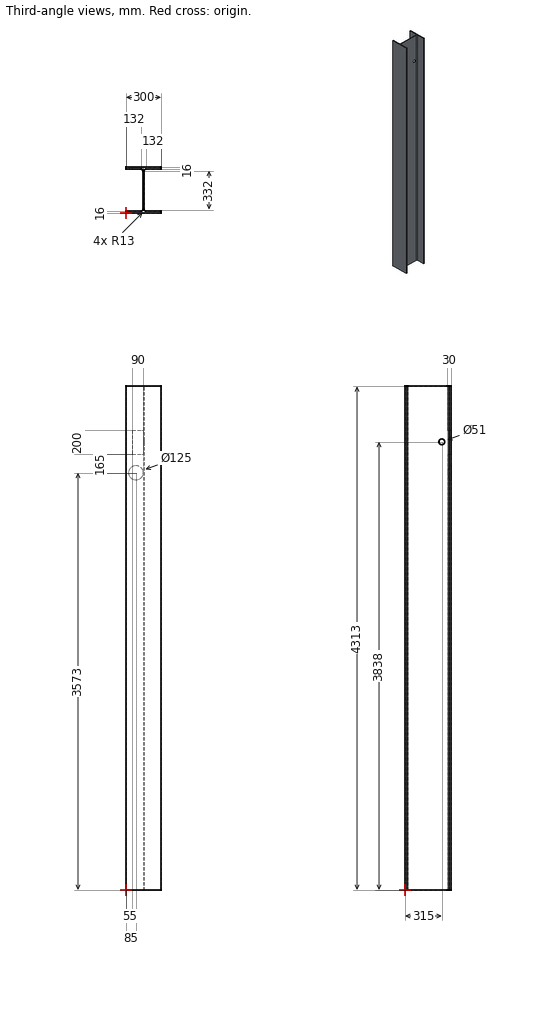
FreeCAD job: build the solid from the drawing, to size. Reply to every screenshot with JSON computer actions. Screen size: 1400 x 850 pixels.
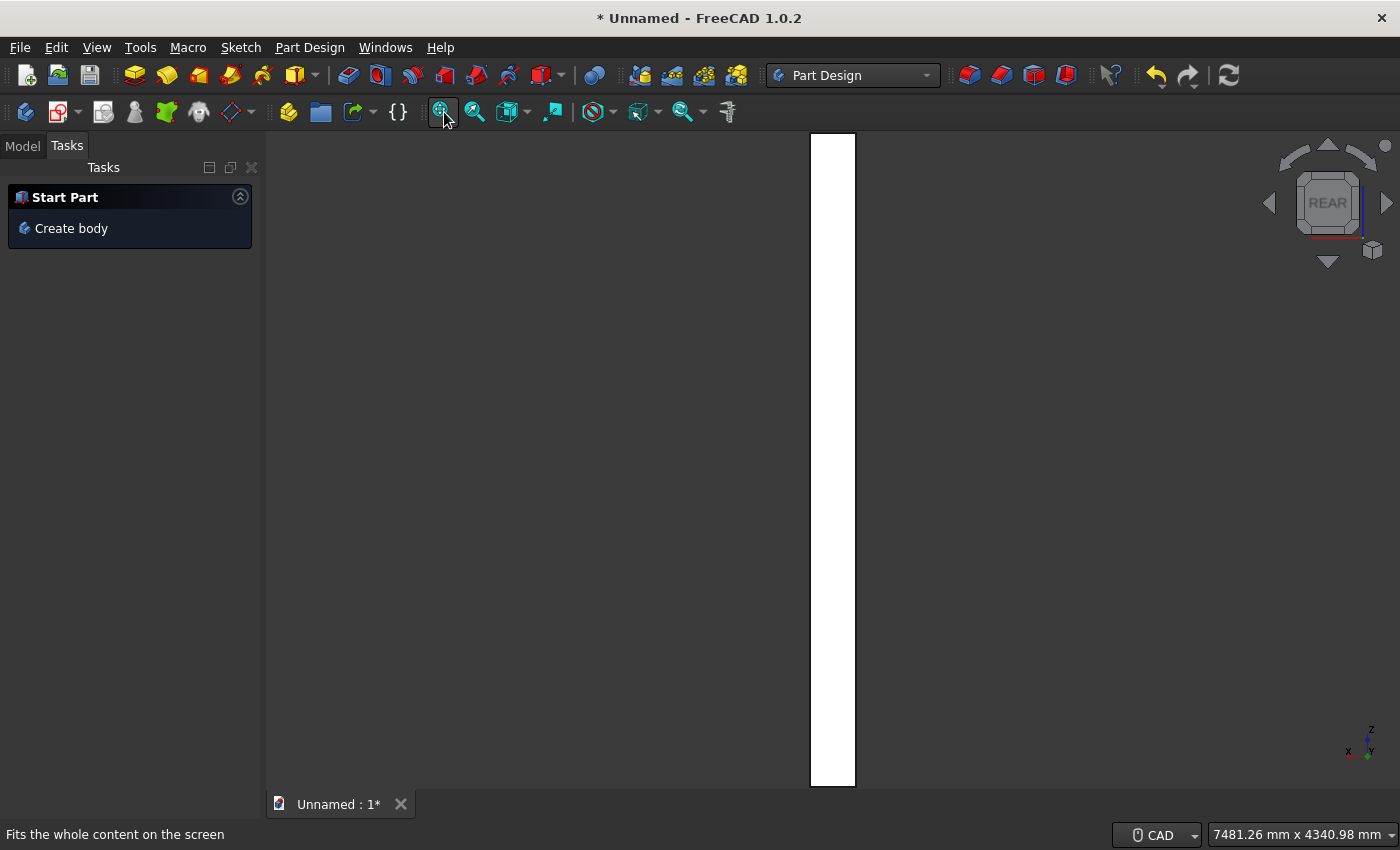
{"action": "left_click", "coordinate": [833, 179]}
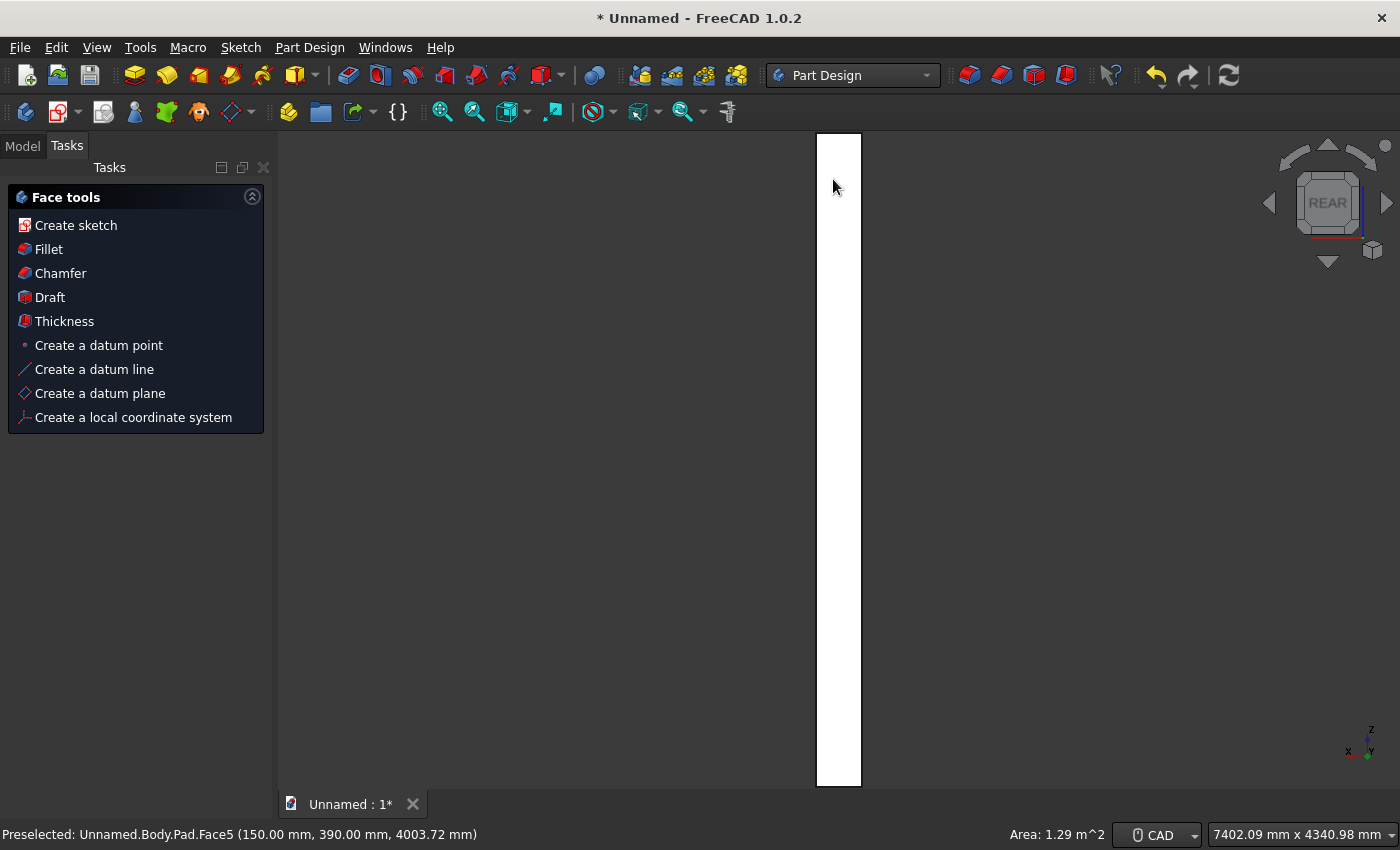
{"action": "left_click", "coordinate": [58, 112]}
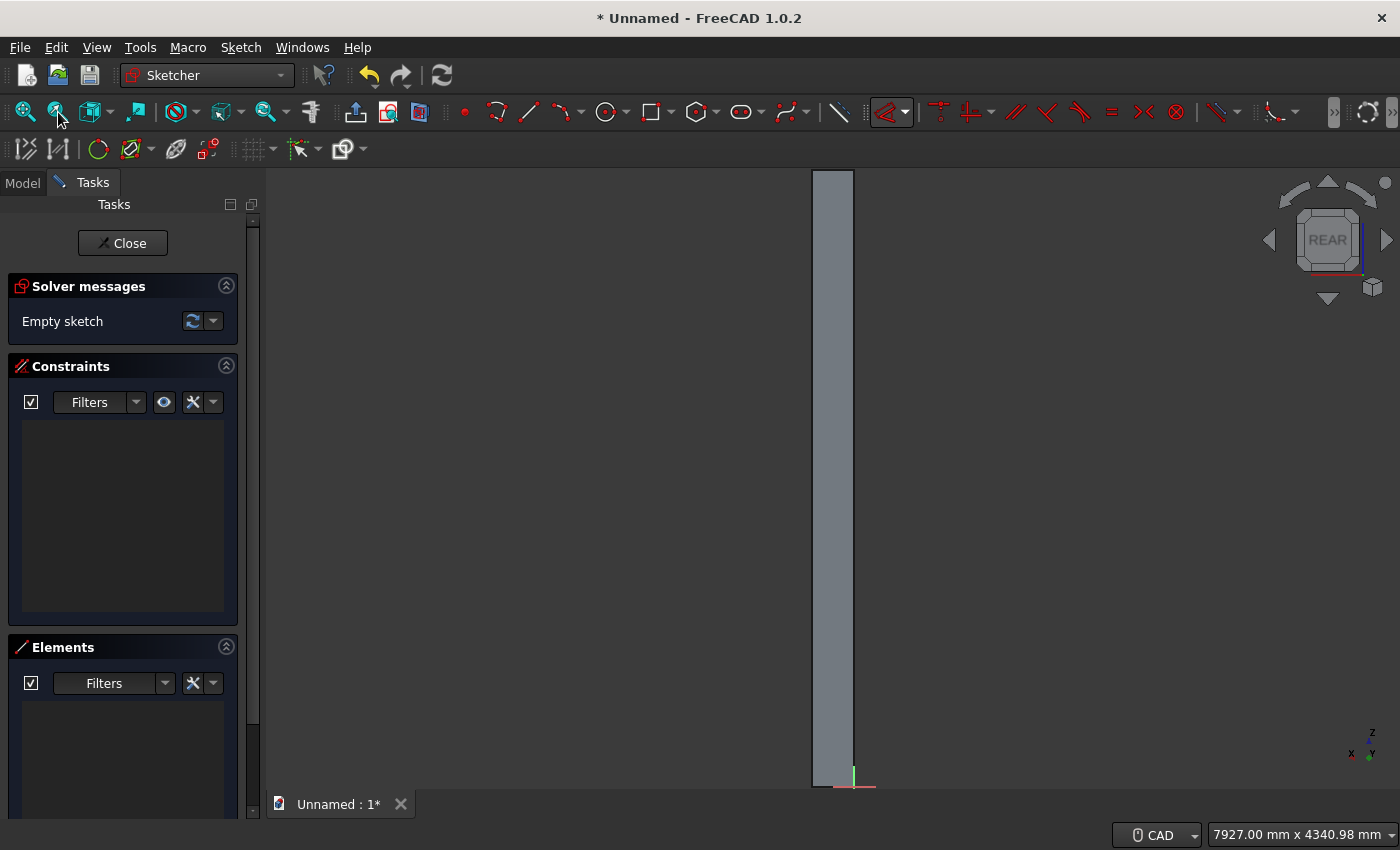
{"action": "scroll", "coordinate": [858, 210], "scroll_direction": "up", "scroll_amount": 9}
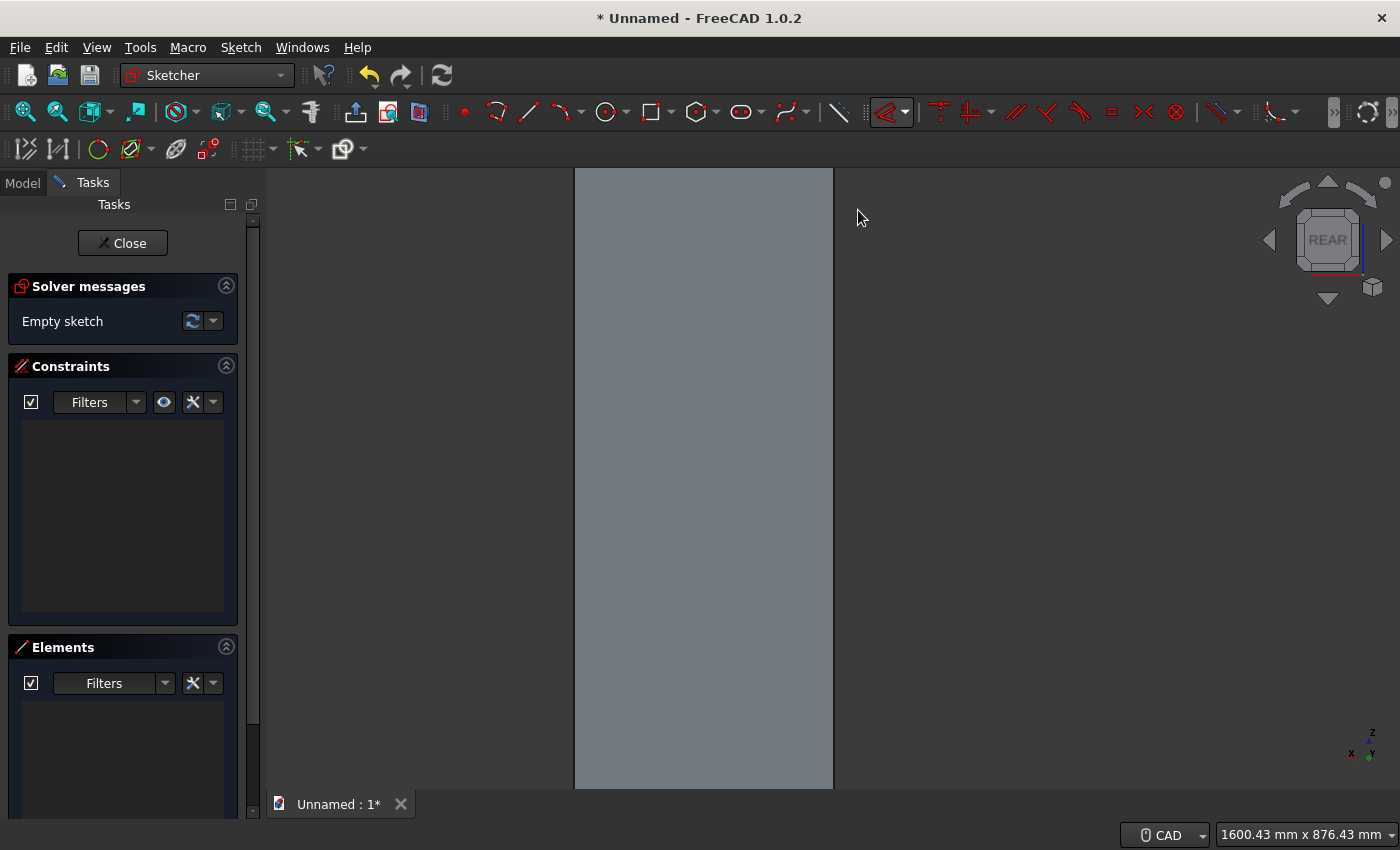
{"action": "left_click", "coordinate": [652, 112]}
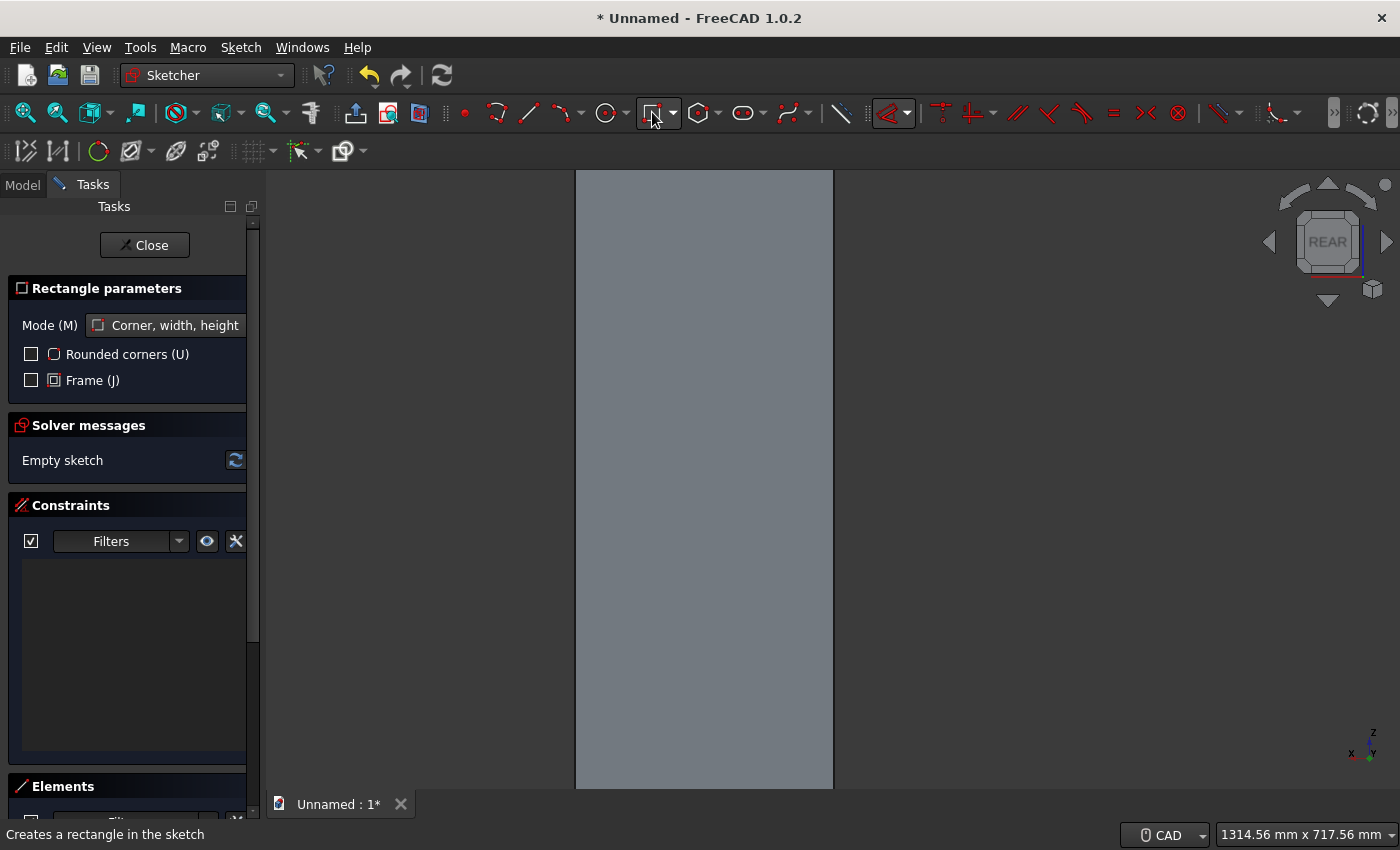
{"action": "left_click", "coordinate": [709, 294]}
{"action": "mouse_move", "coordinate": [786, 466]}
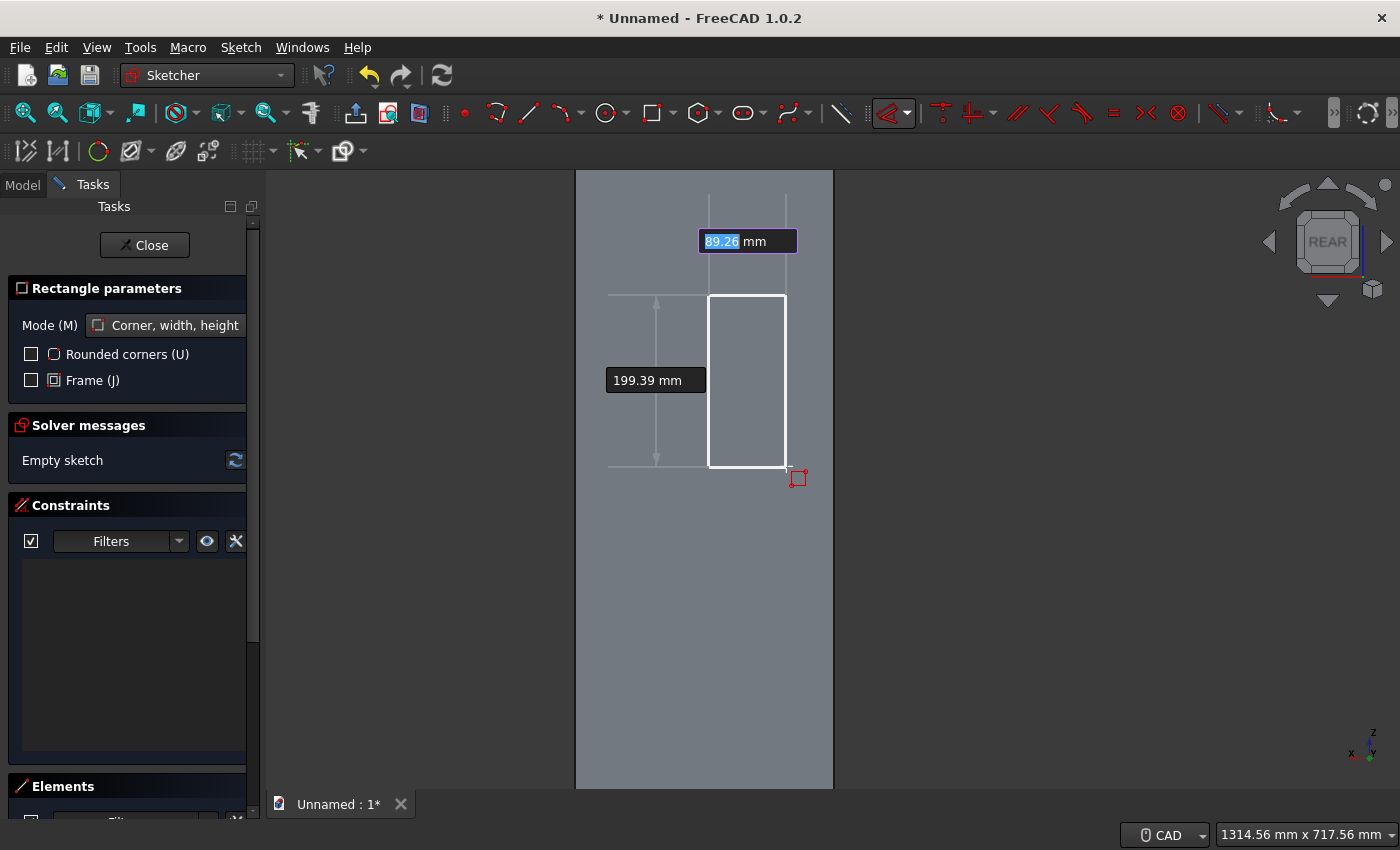
{"action": "type", "text": "90"}
{"action": "key", "text": "Tab"}
{"action": "type", "text": "200"}
{"action": "key", "text": "Return"}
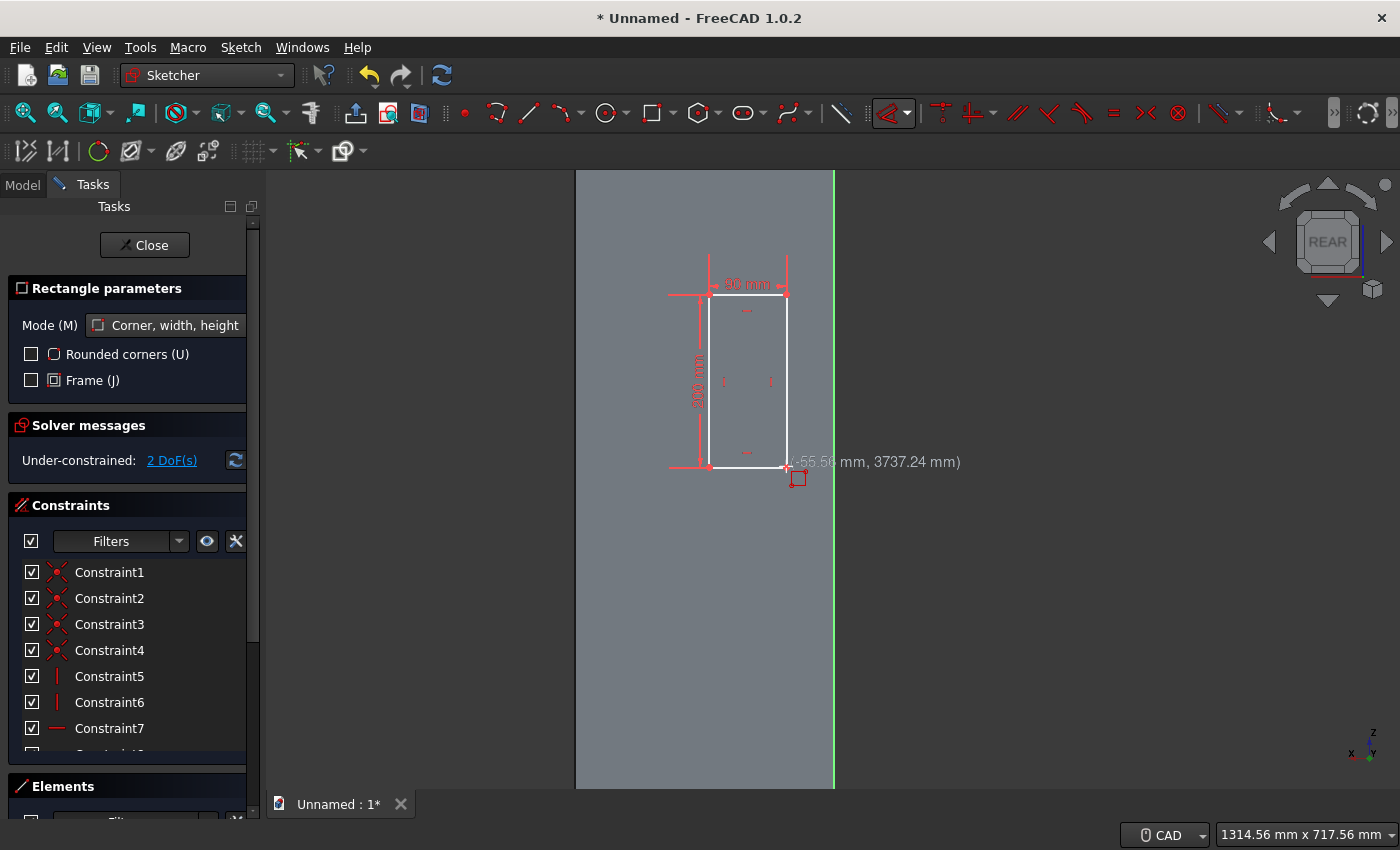
{"action": "left_click", "coordinate": [606, 114]}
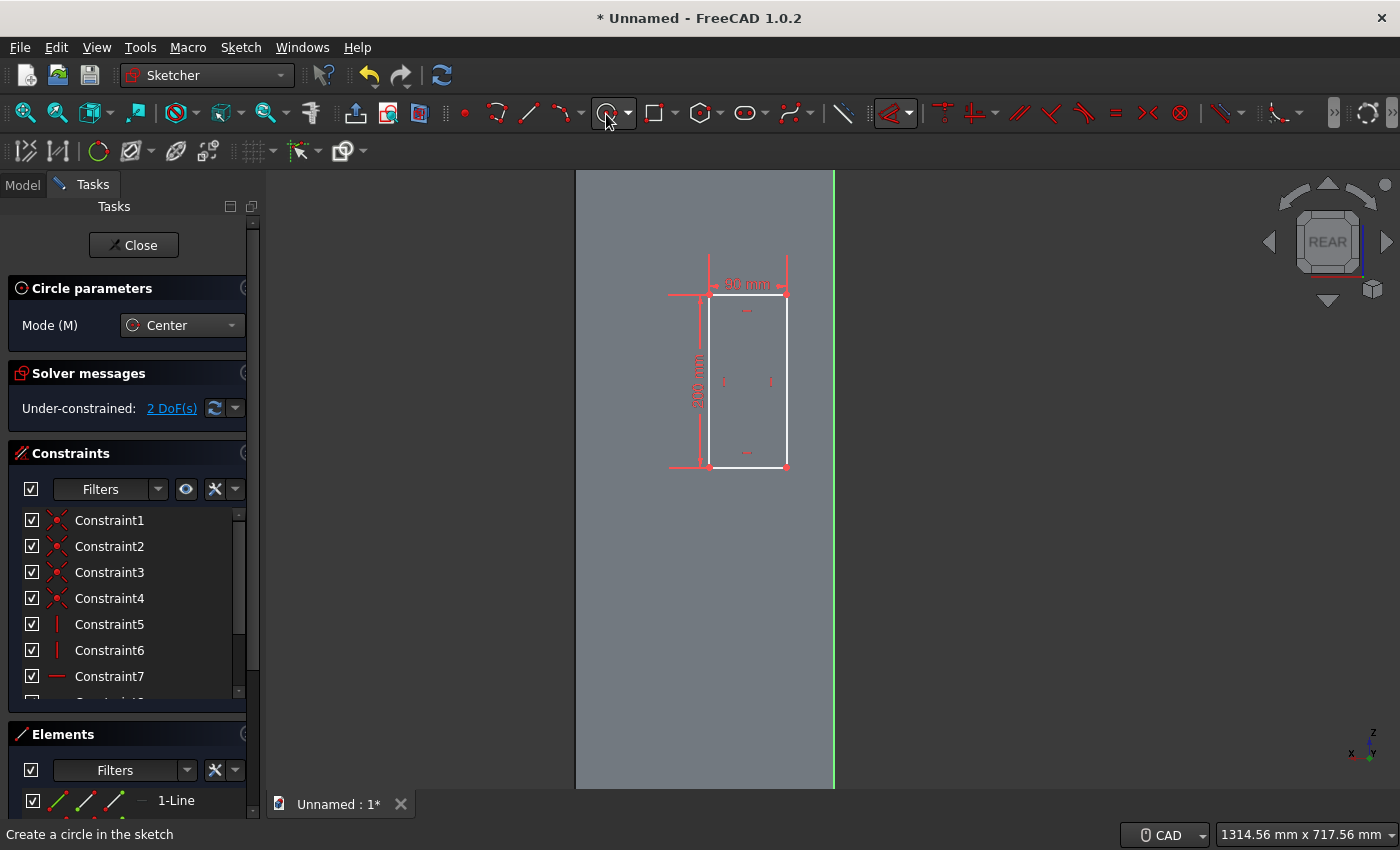
{"action": "left_click", "coordinate": [761, 609]}
{"action": "mouse_move", "coordinate": [799, 571]}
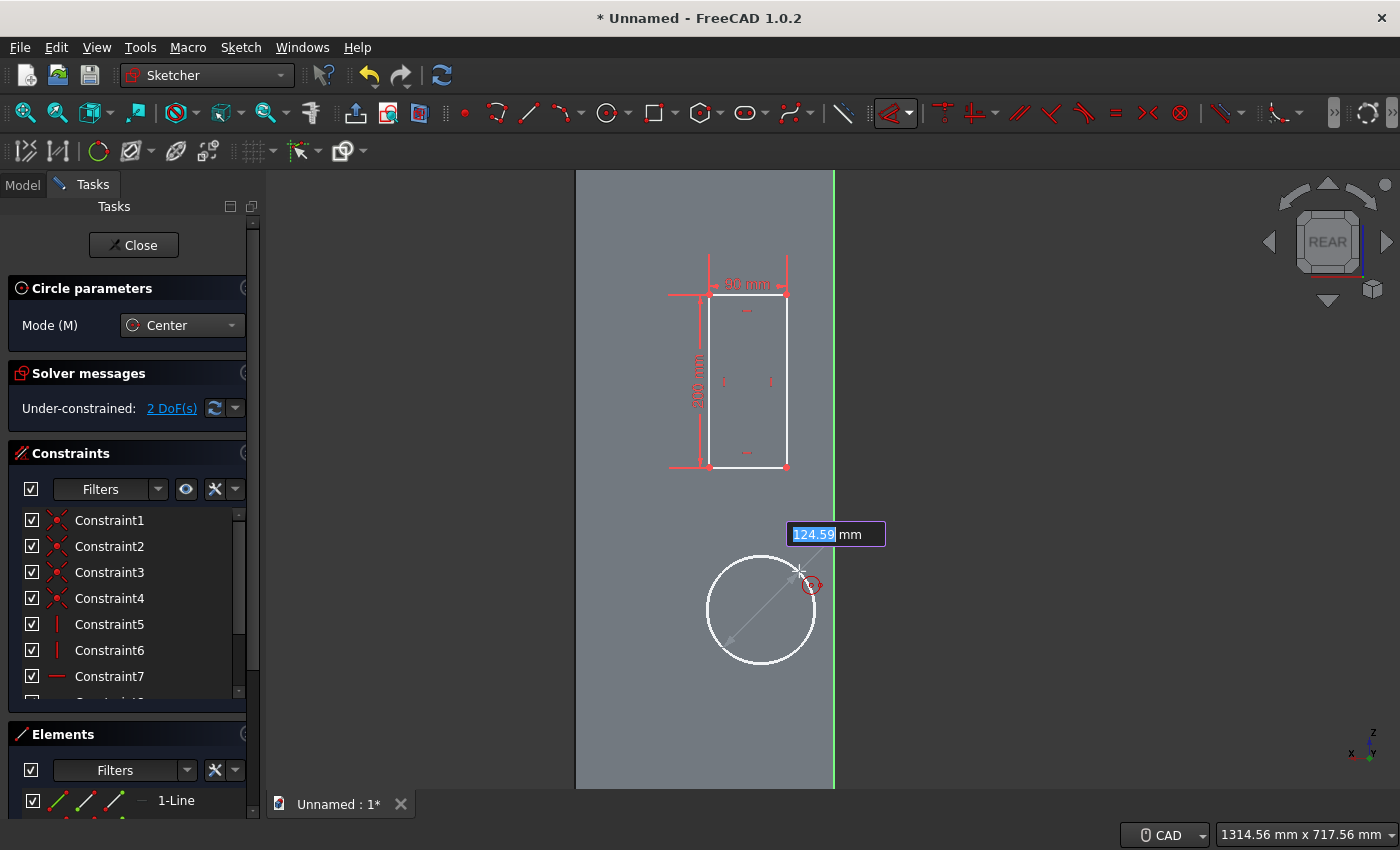
{"action": "type", "text": "125"}
{"action": "key", "text": "Return"}
{"action": "key", "text": "Escape"}